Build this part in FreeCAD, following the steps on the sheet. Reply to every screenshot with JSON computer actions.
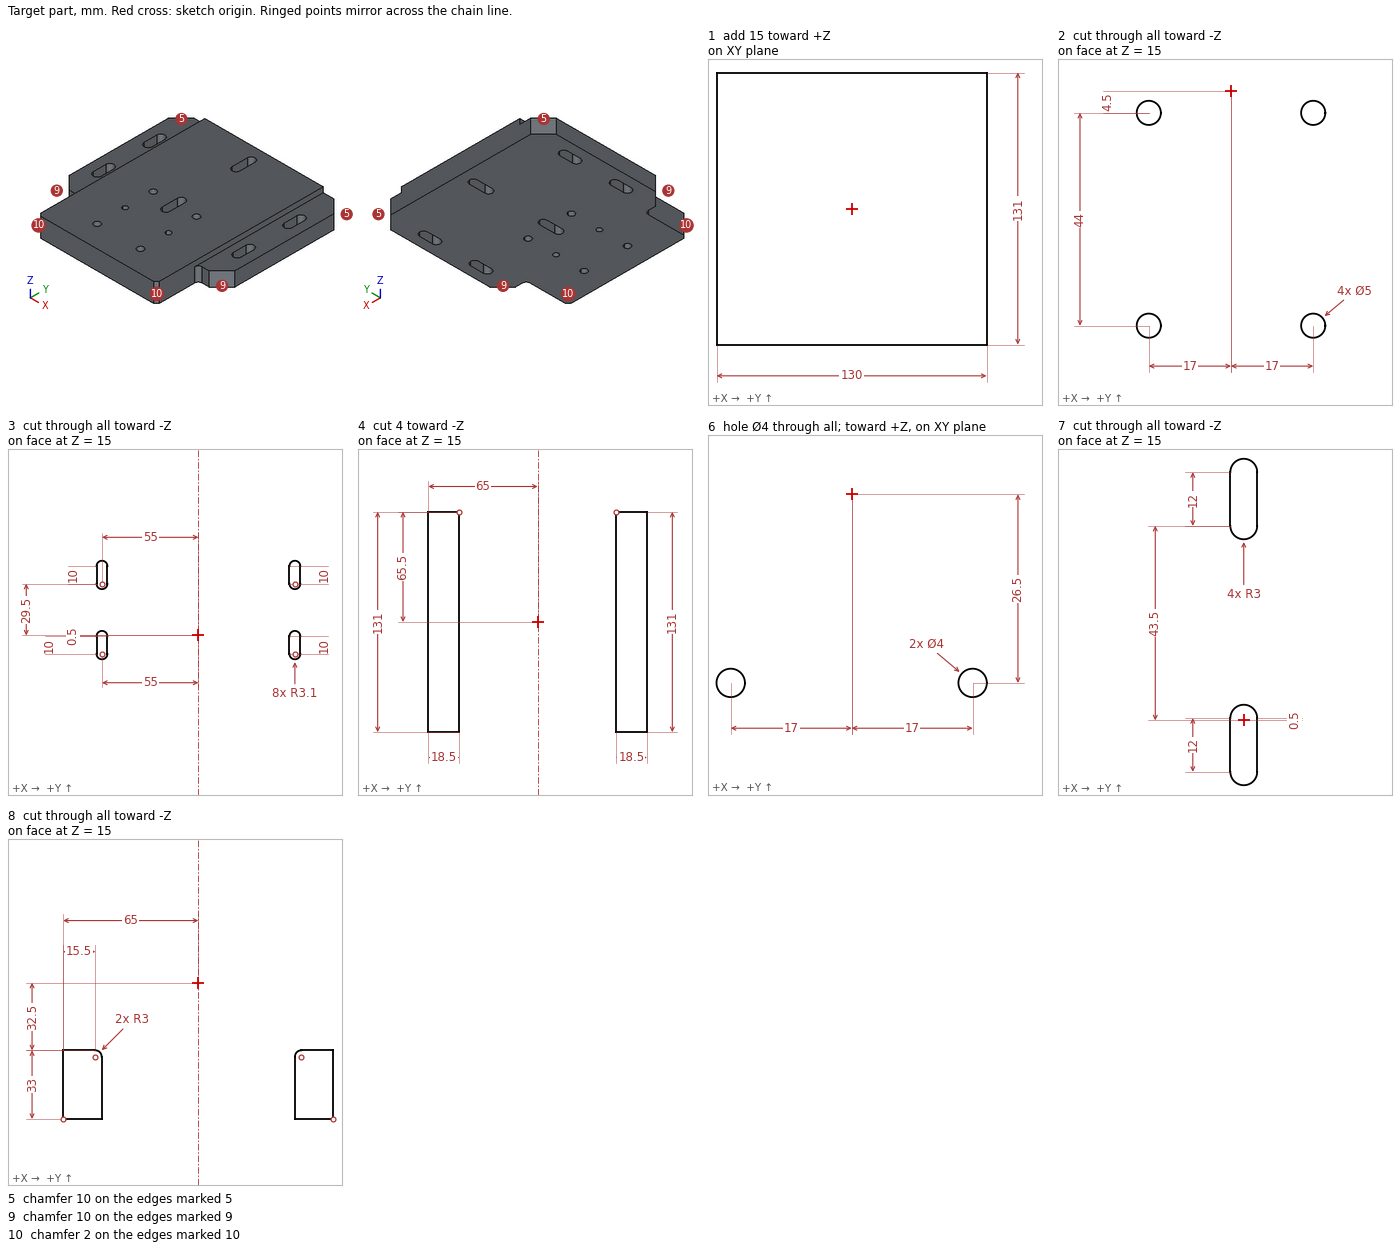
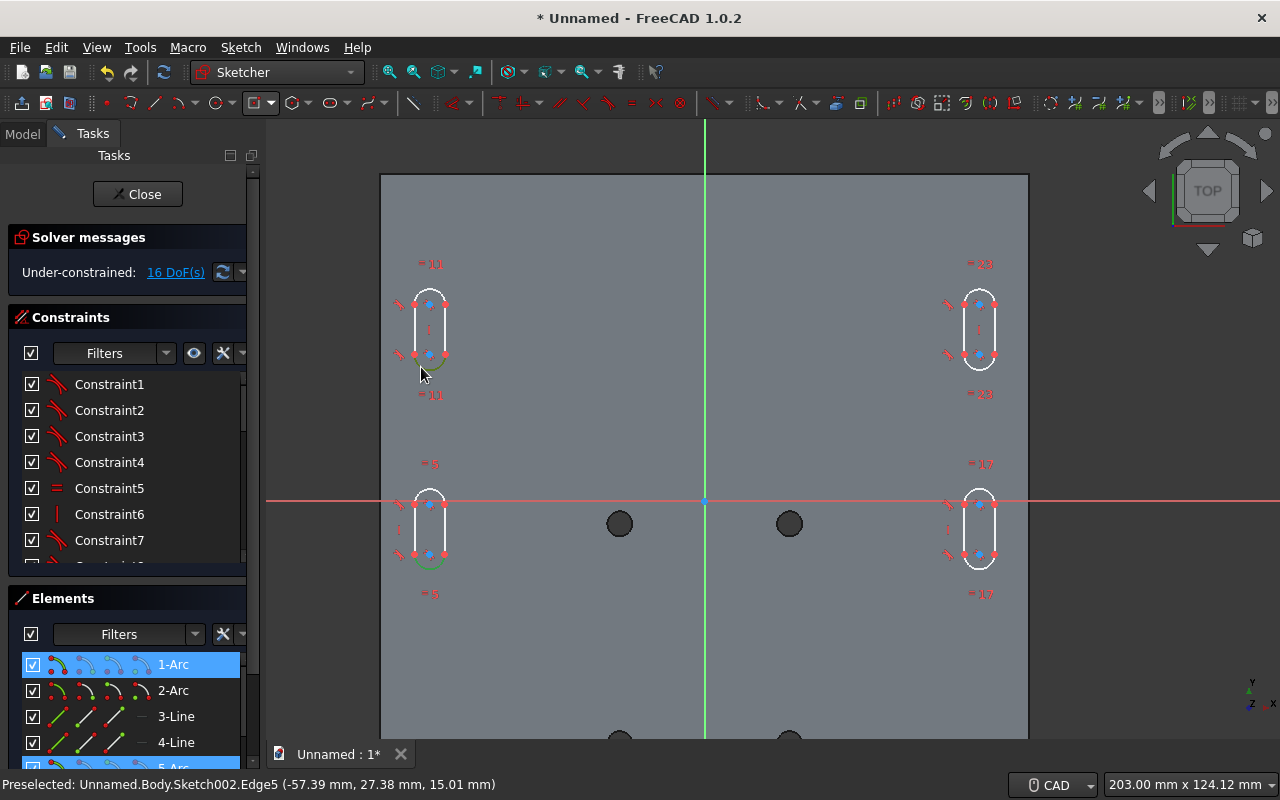
{"action": "left_click", "coordinate": [971, 566]}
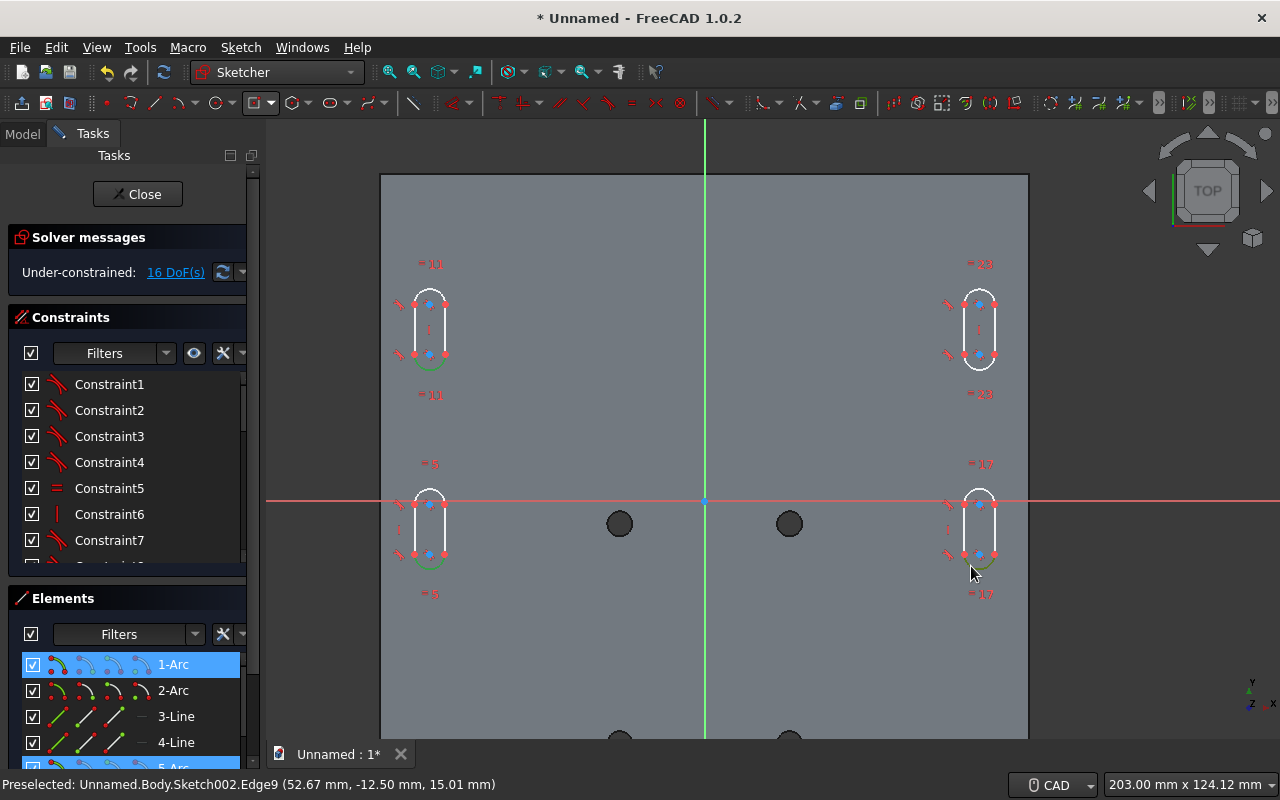
{"action": "left_click", "coordinate": [971, 367]}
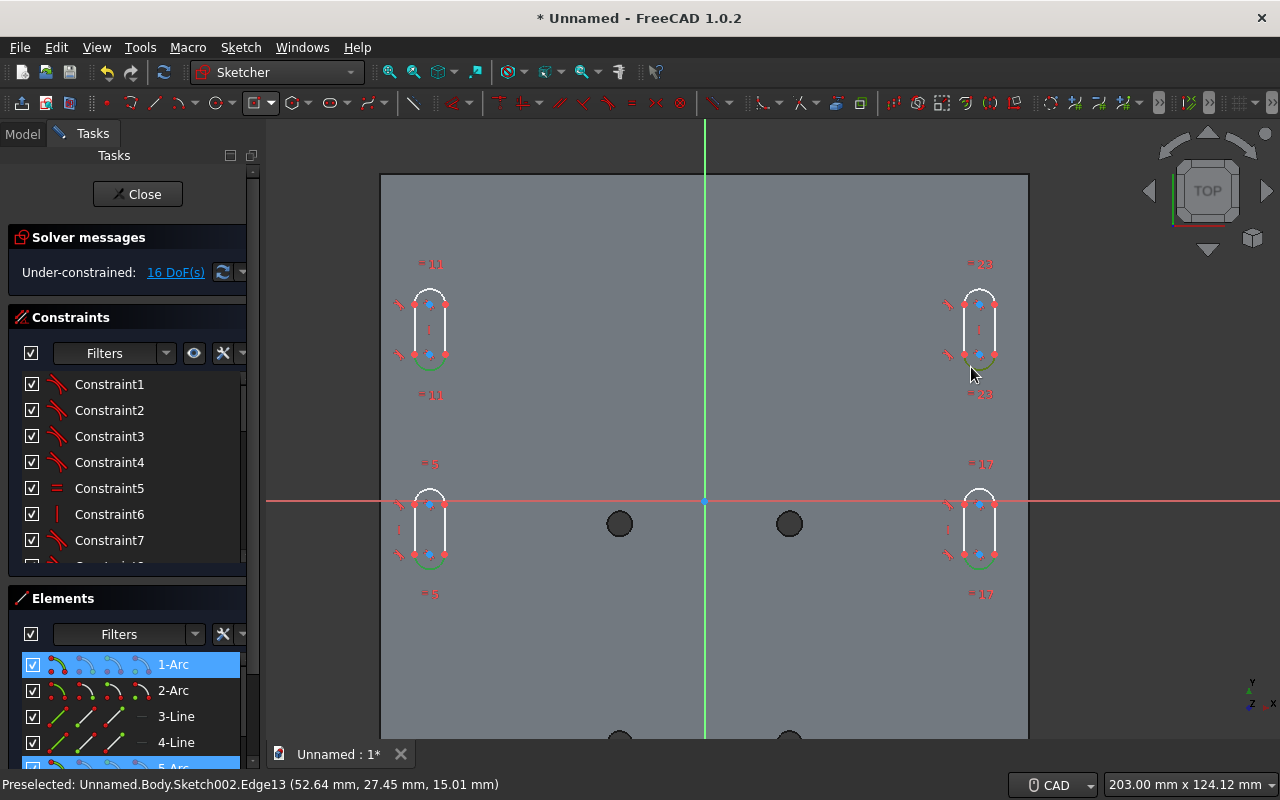
{"action": "key", "text": "e"}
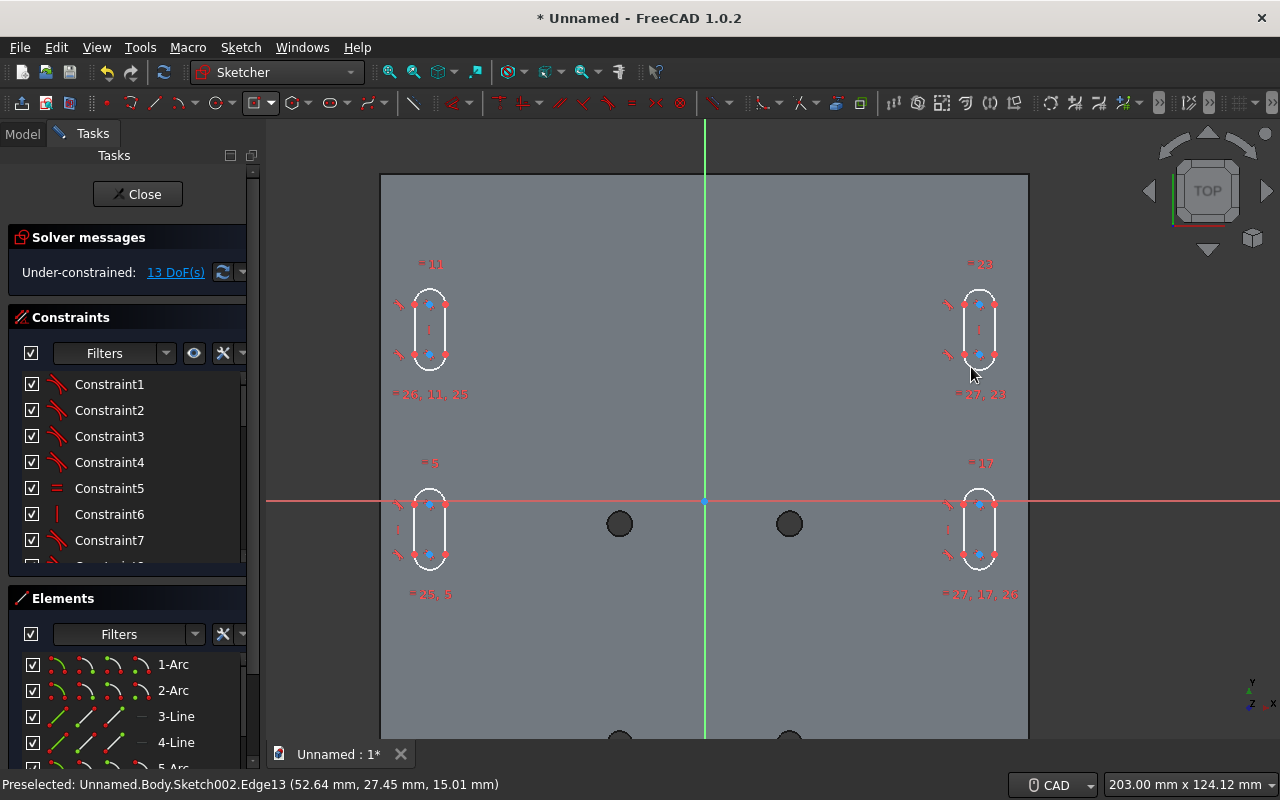
{"action": "left_click", "coordinate": [430, 554]}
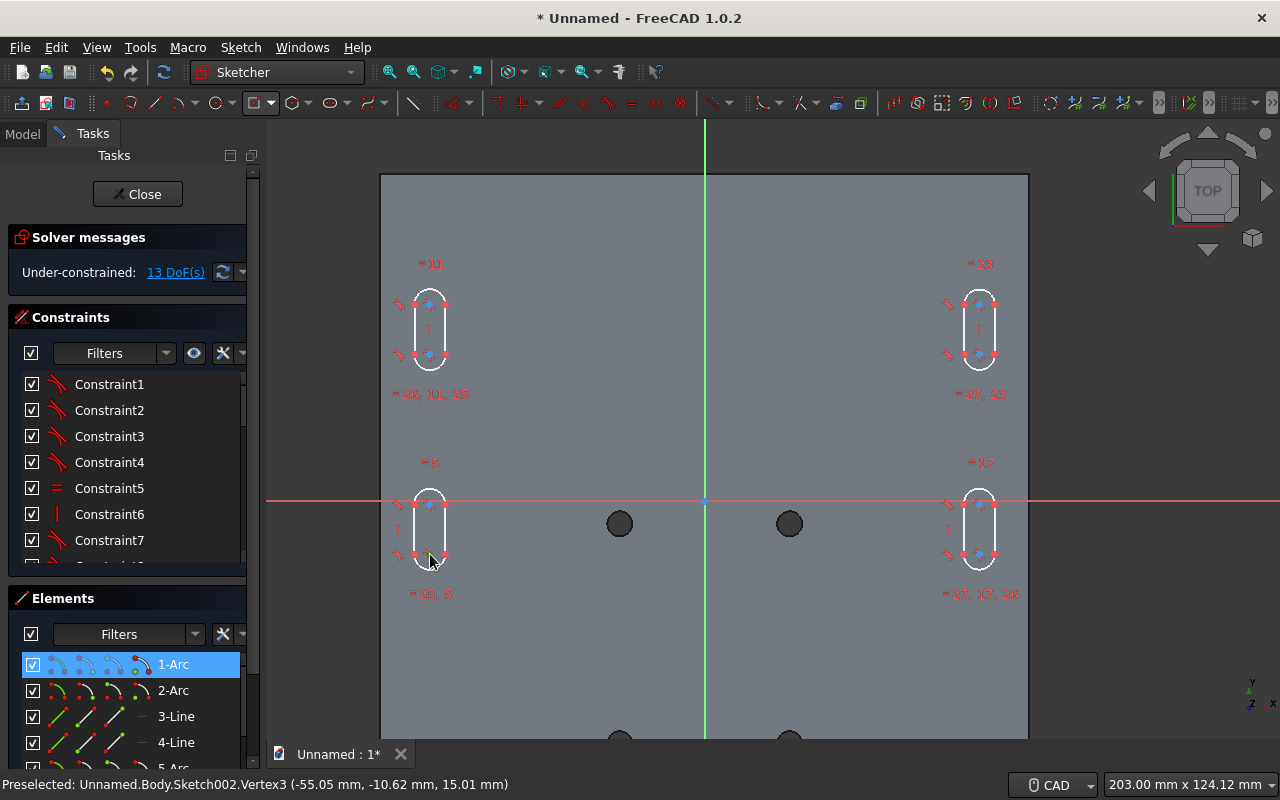
{"action": "left_click", "coordinate": [979, 554]}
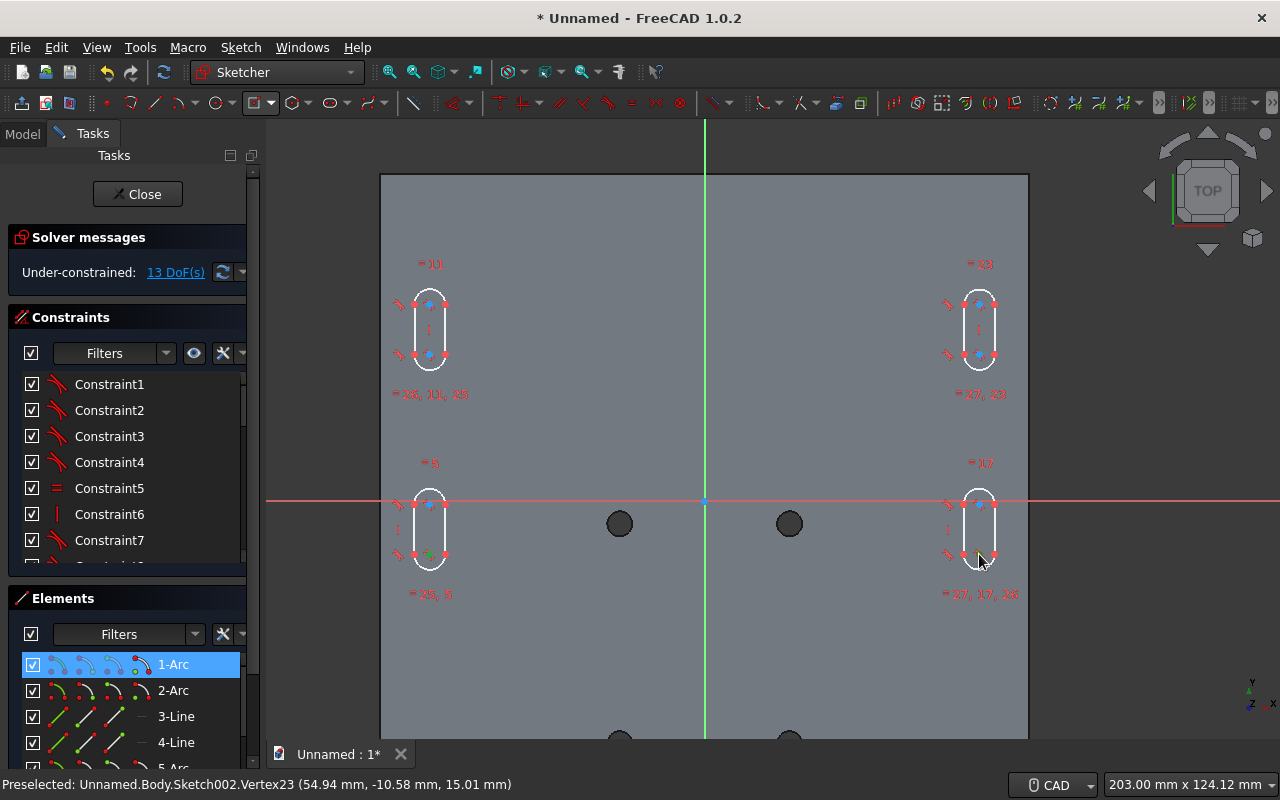
{"action": "left_click", "coordinate": [705, 671]}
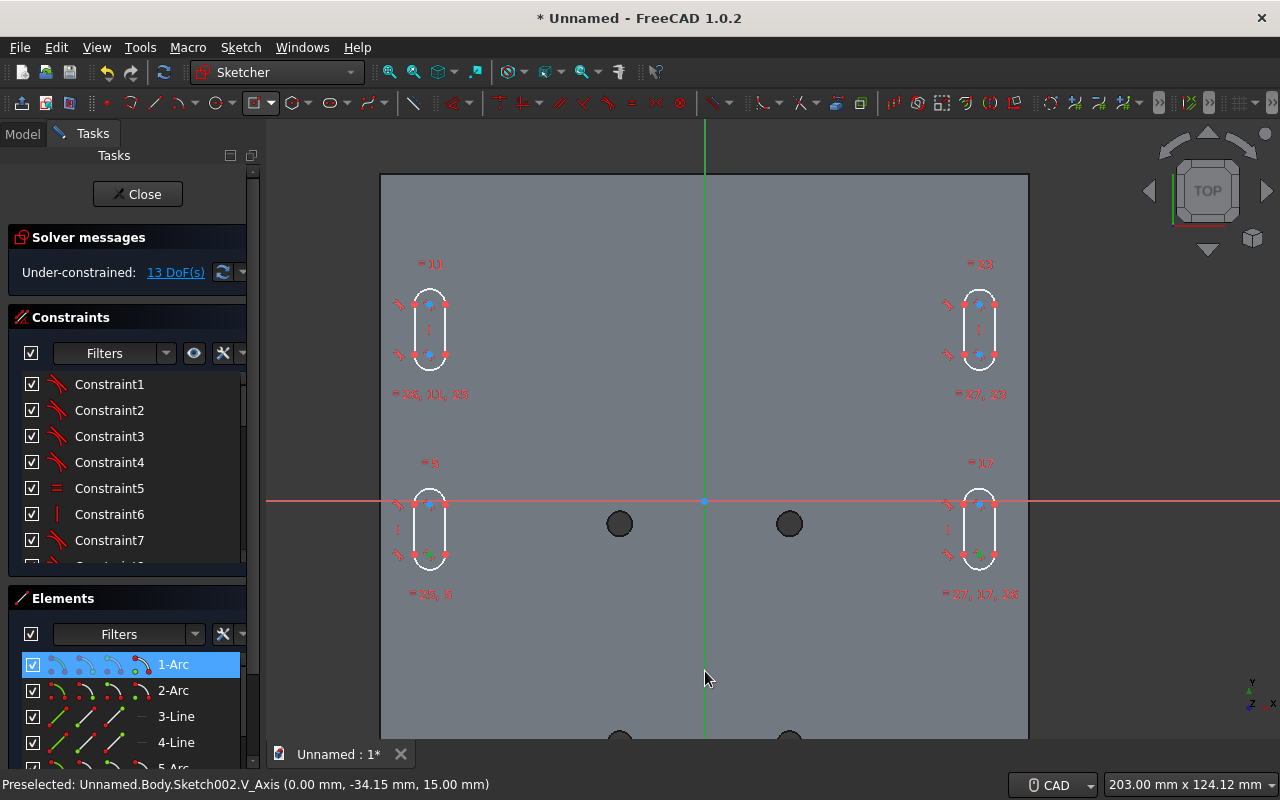
{"action": "key", "text": "s"}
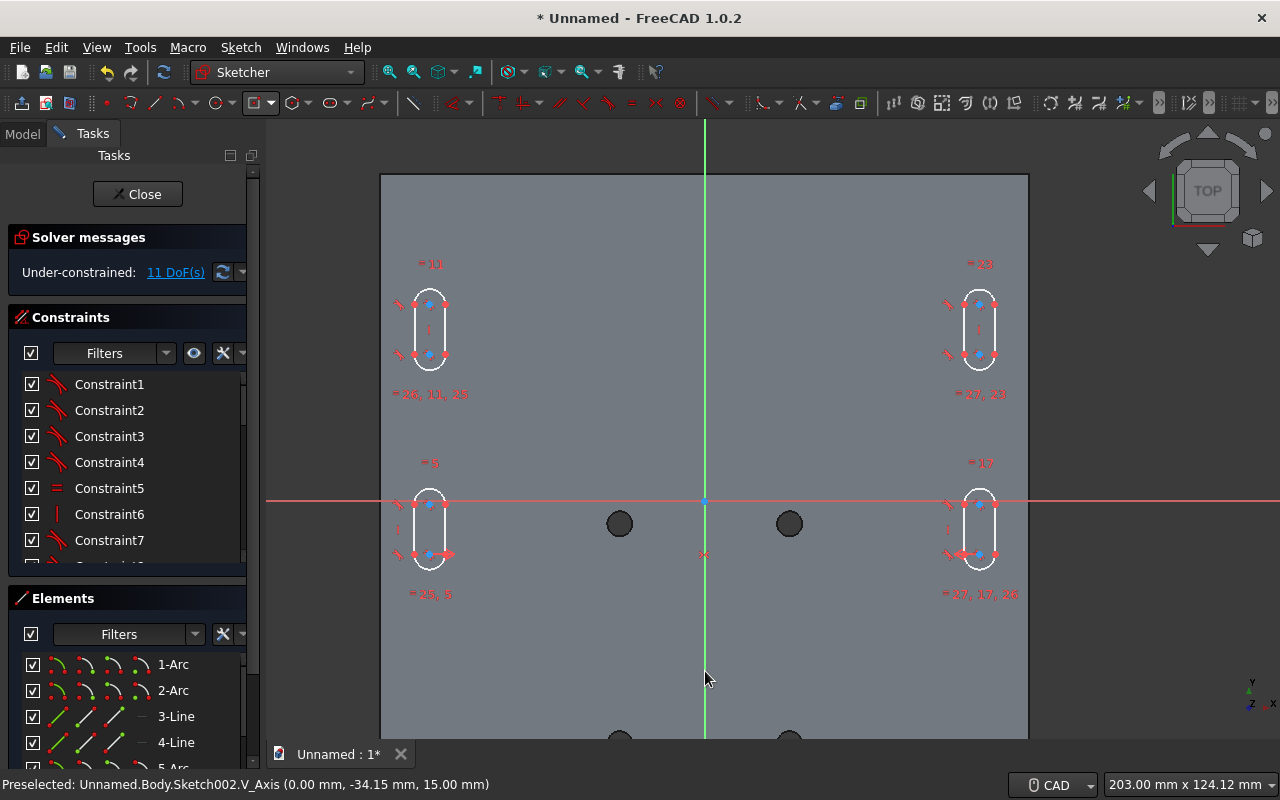
{"action": "left_click", "coordinate": [430, 355]}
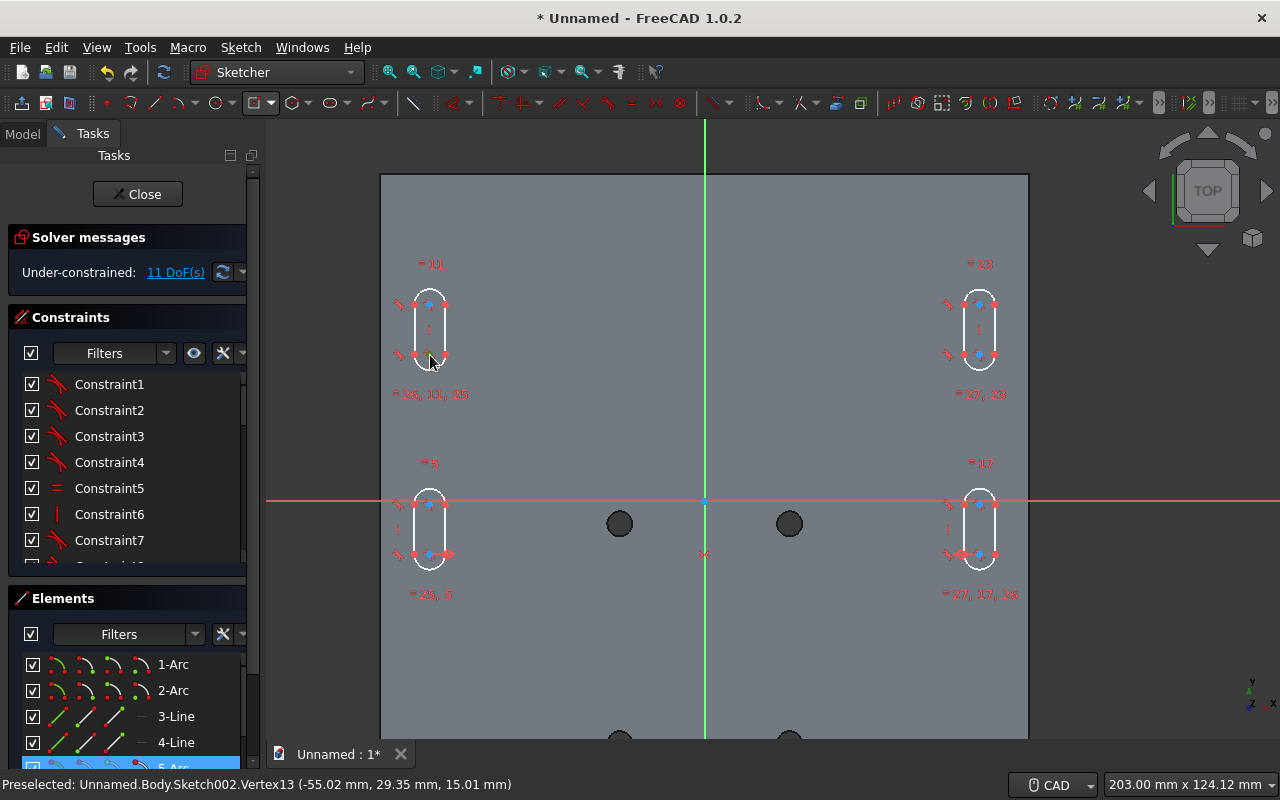
{"action": "left_click", "coordinate": [980, 354]}